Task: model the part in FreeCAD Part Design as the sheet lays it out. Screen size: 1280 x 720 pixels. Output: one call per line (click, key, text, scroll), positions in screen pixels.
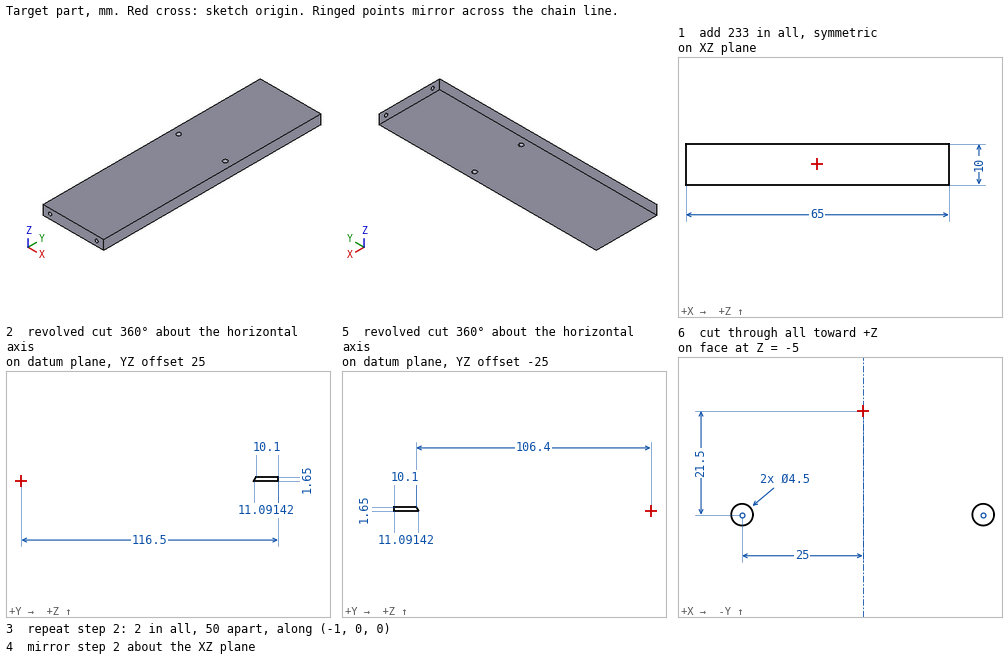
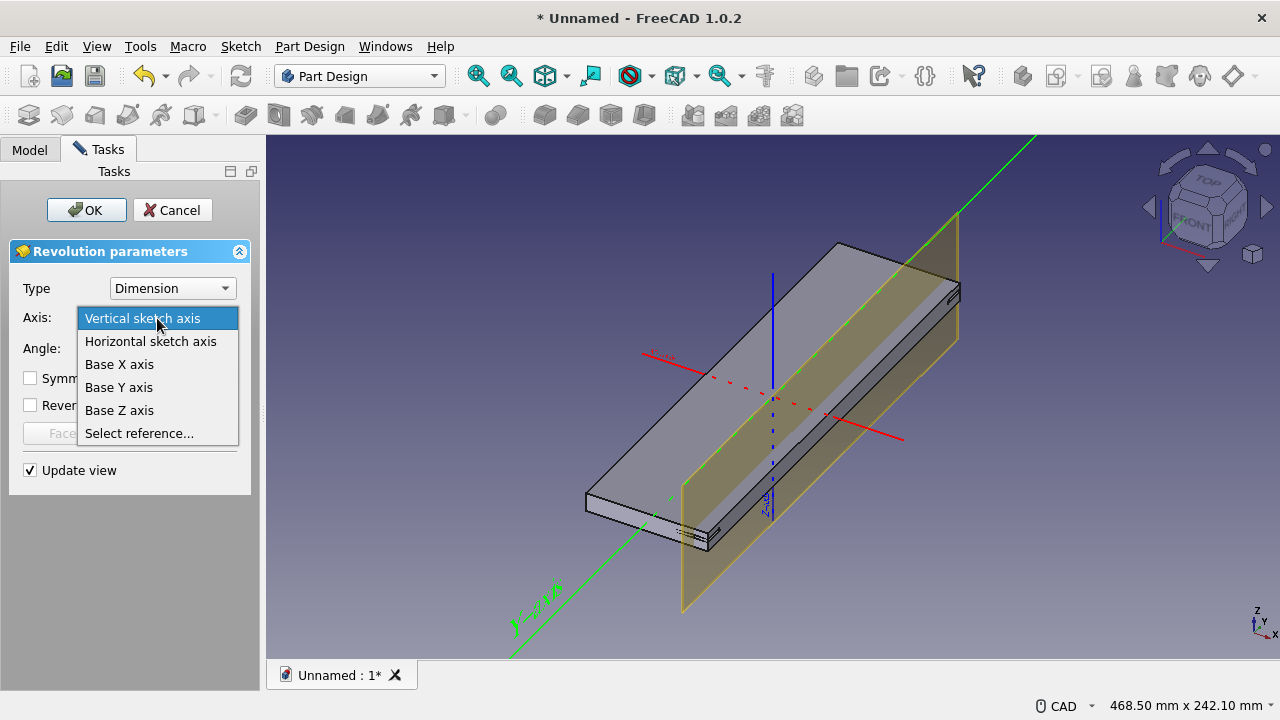
click(156, 342)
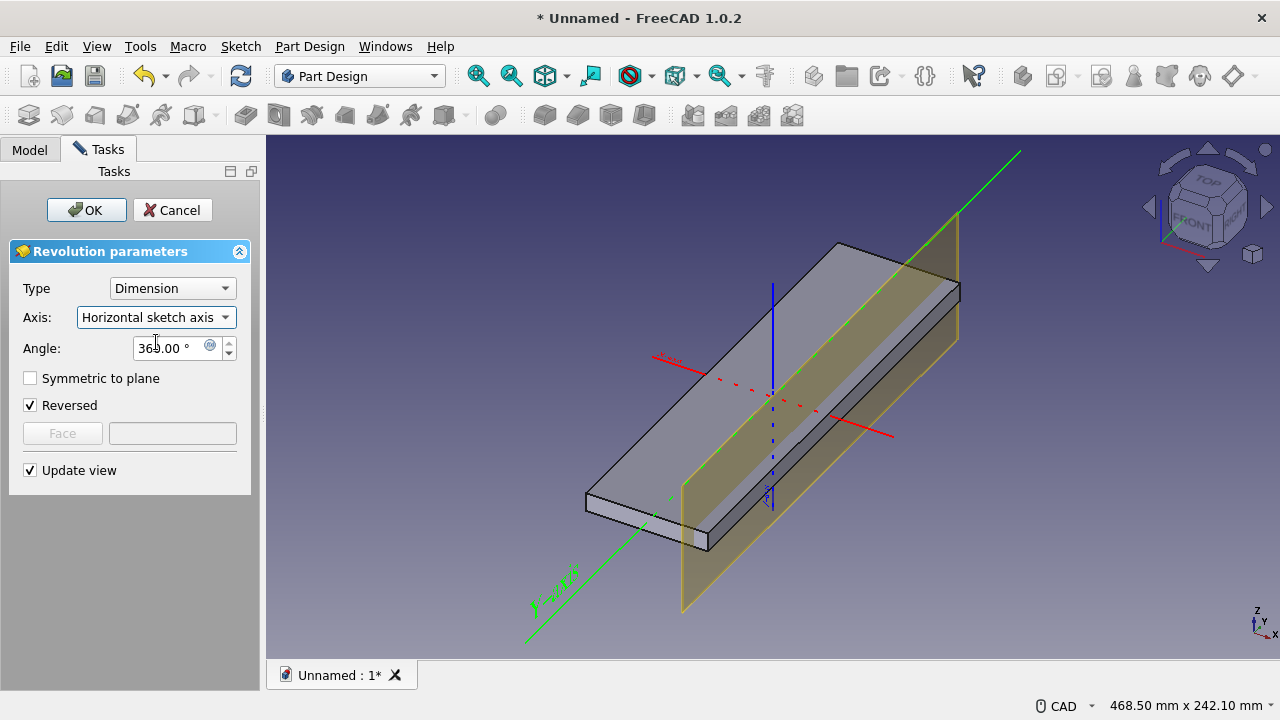
click(87, 210)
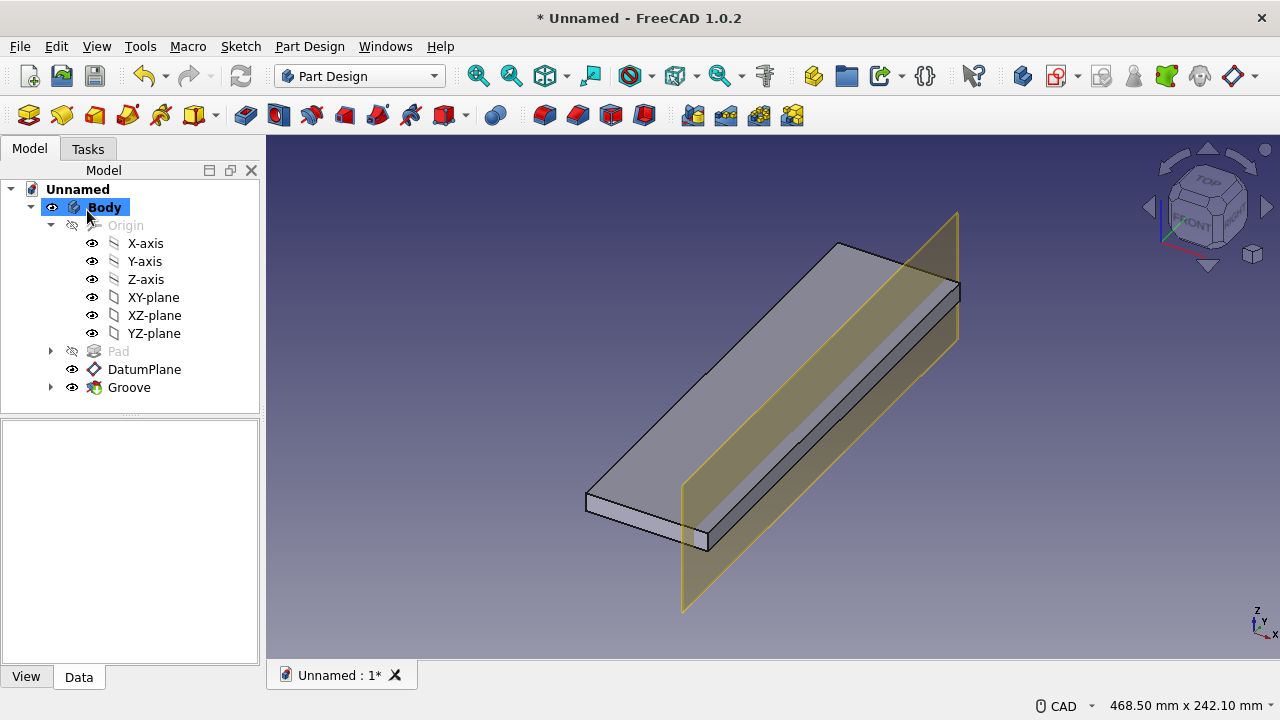
click(117, 369)
key(space)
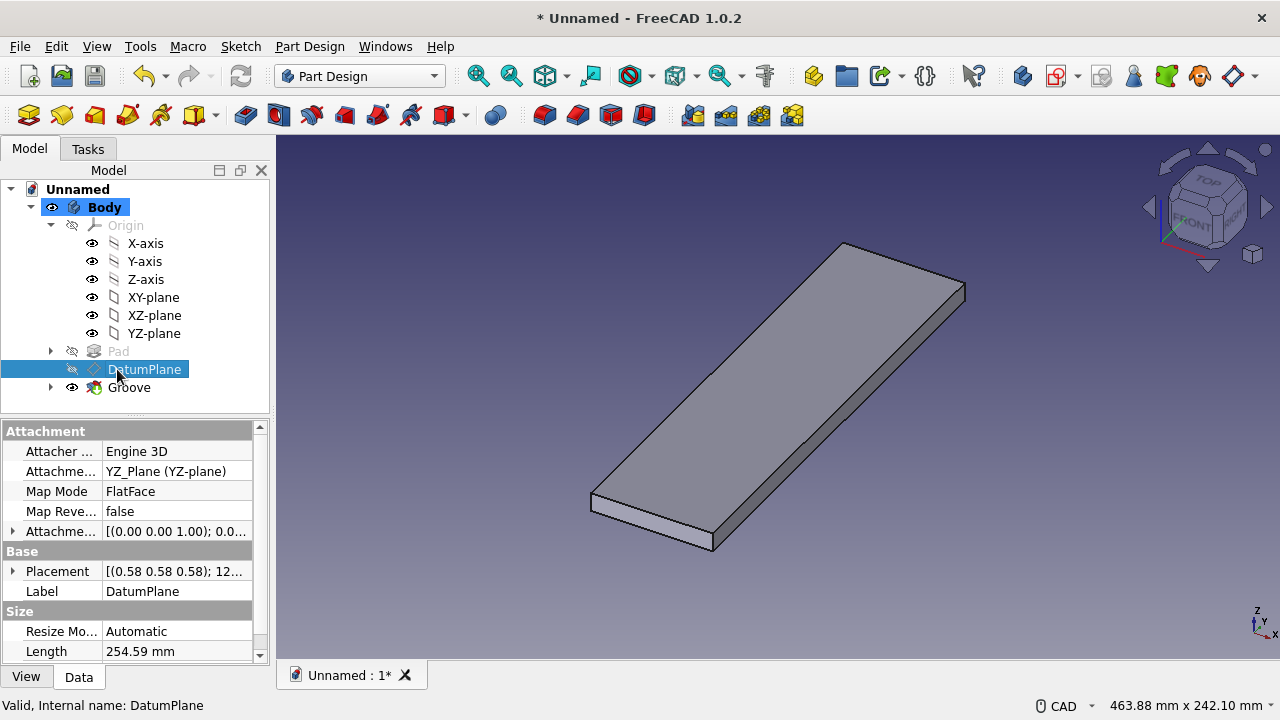
click(117, 387)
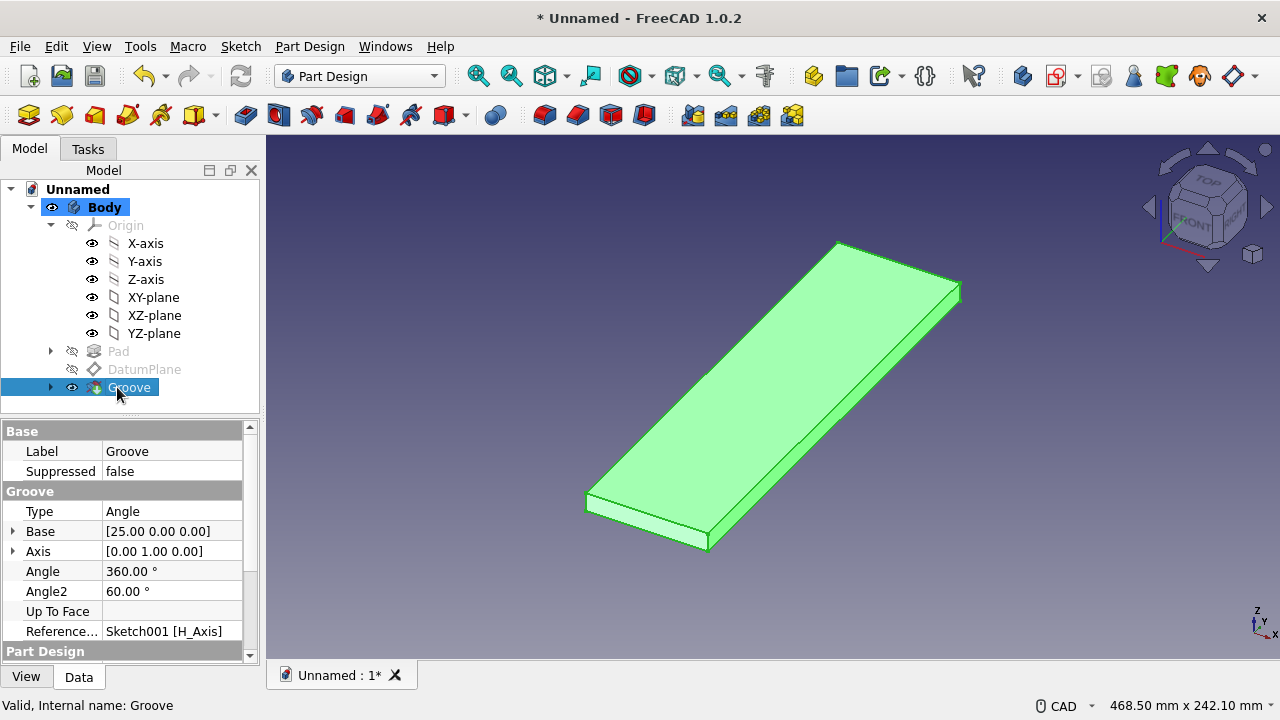
click(726, 116)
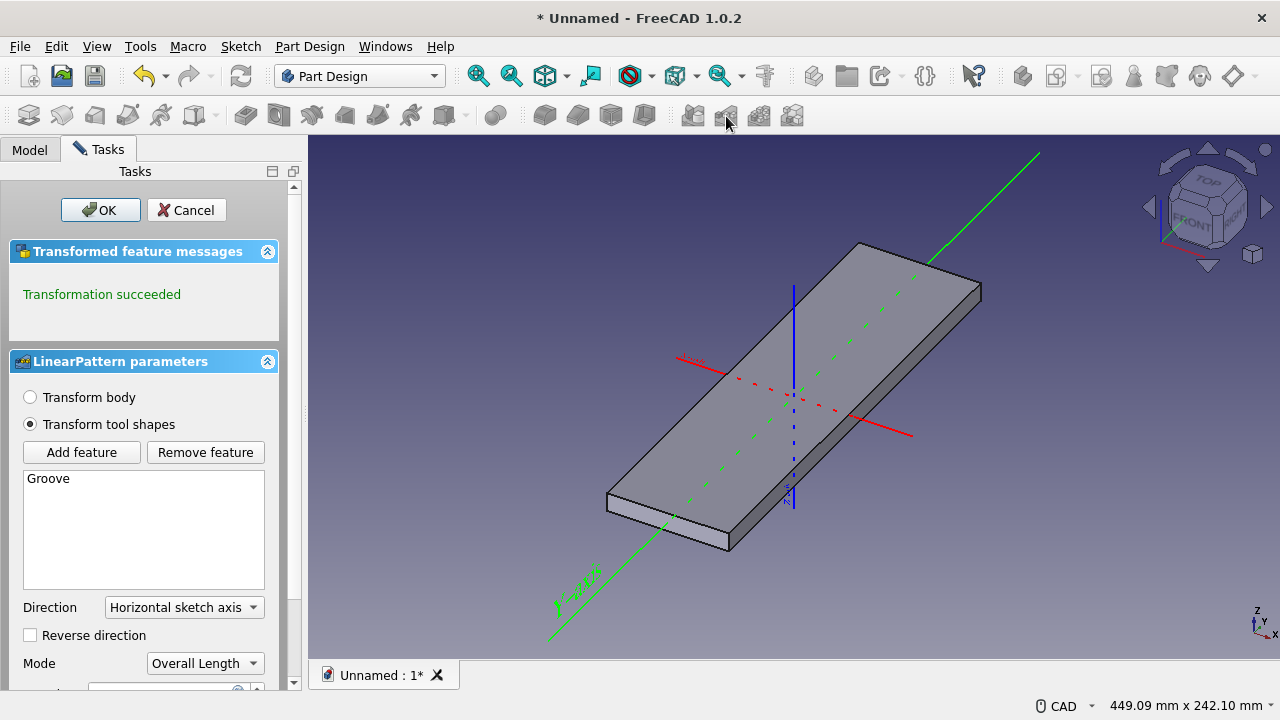
click(185, 608)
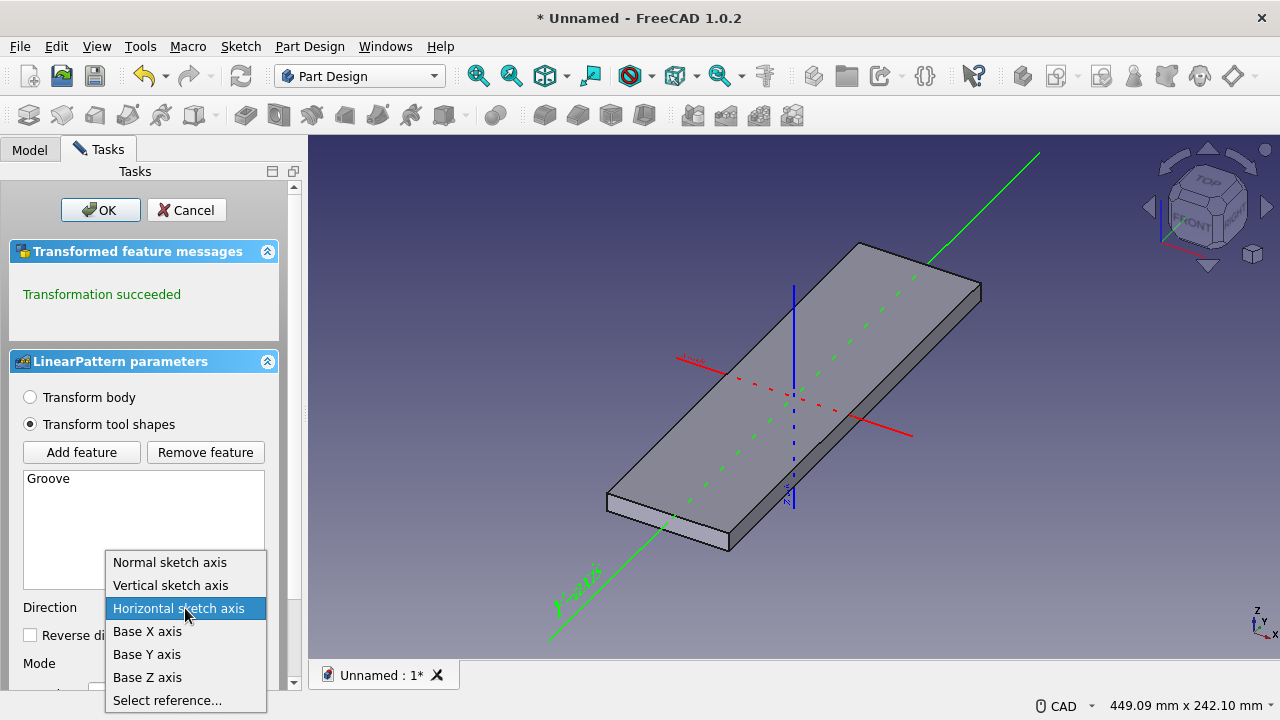
click(184, 632)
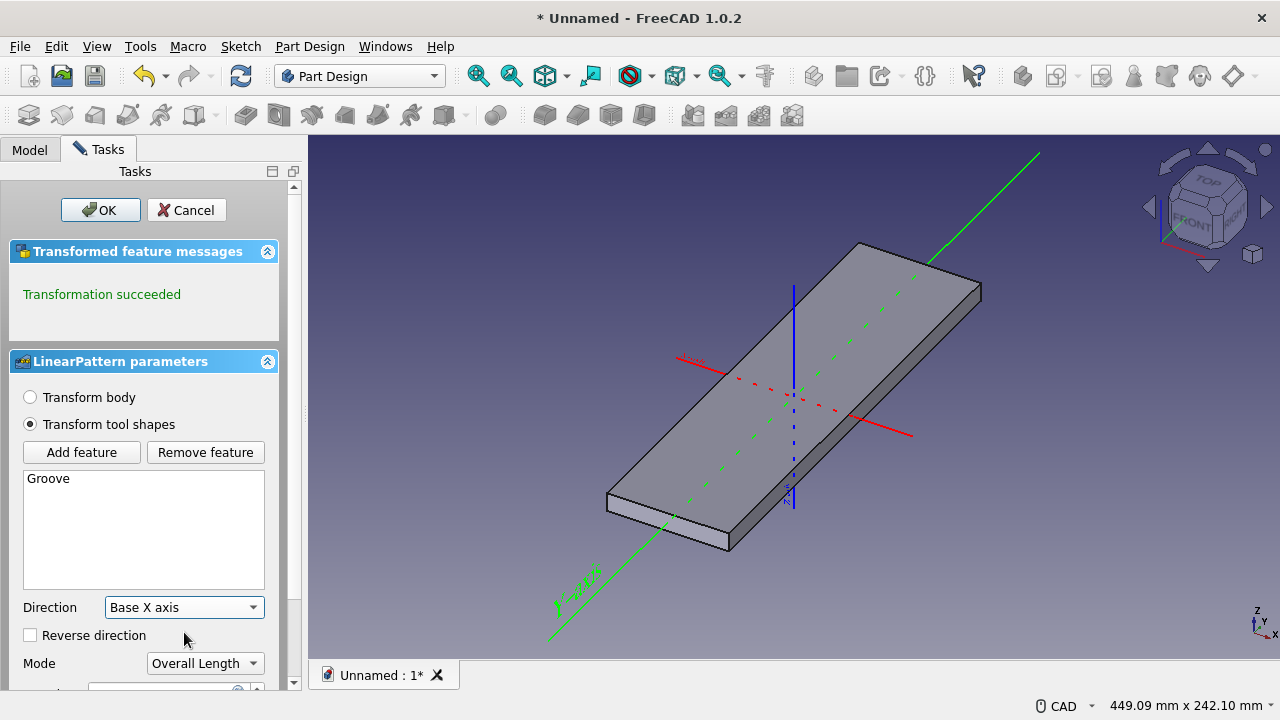
click(206, 664)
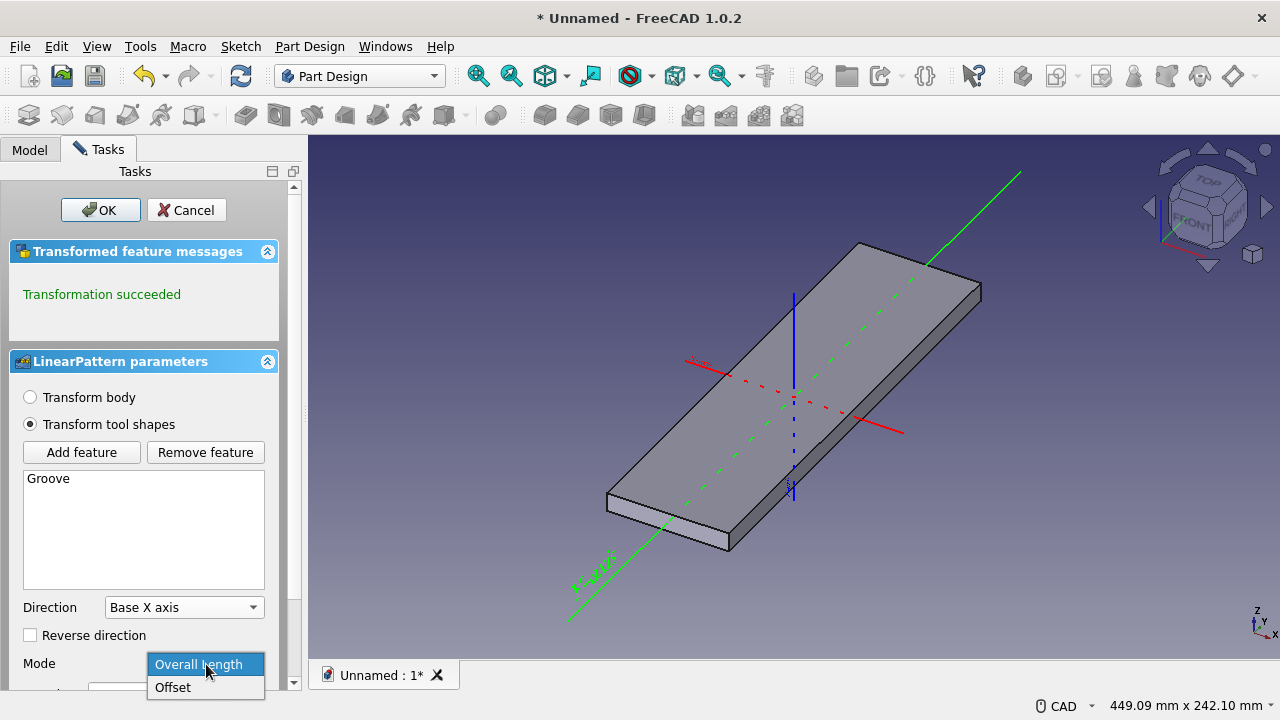
click(204, 688)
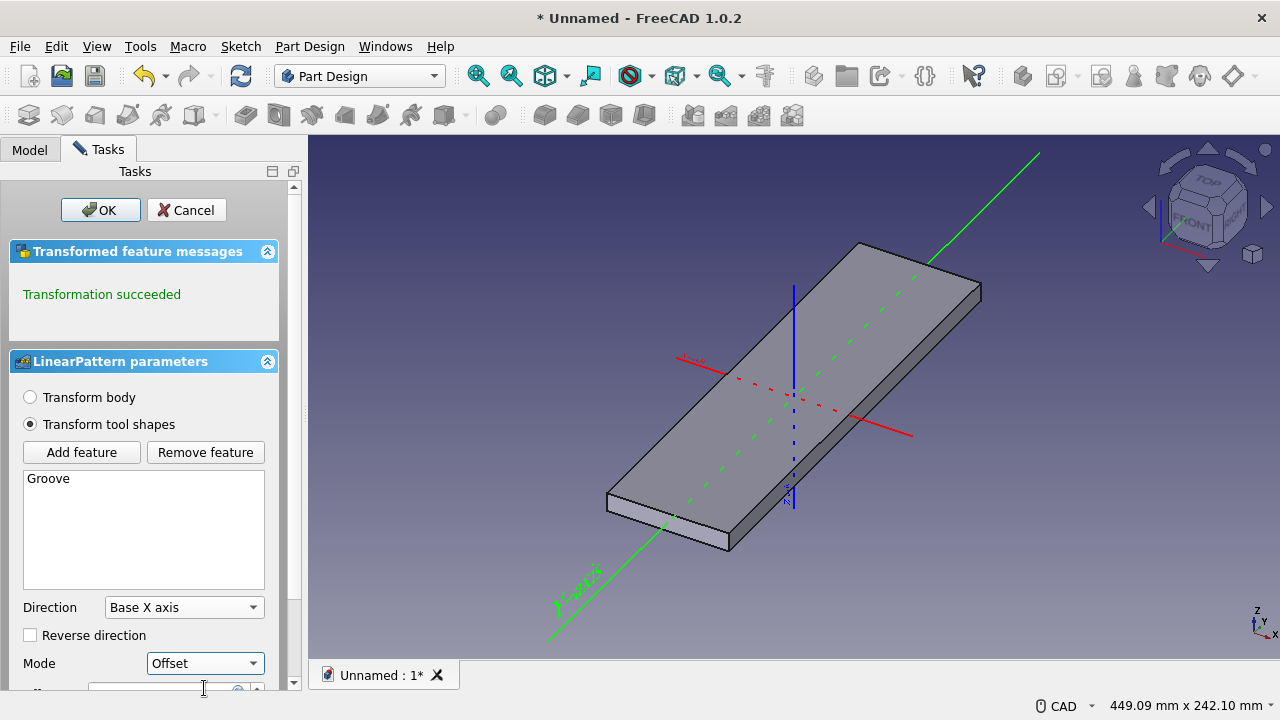
scroll(294, 436, down, 2)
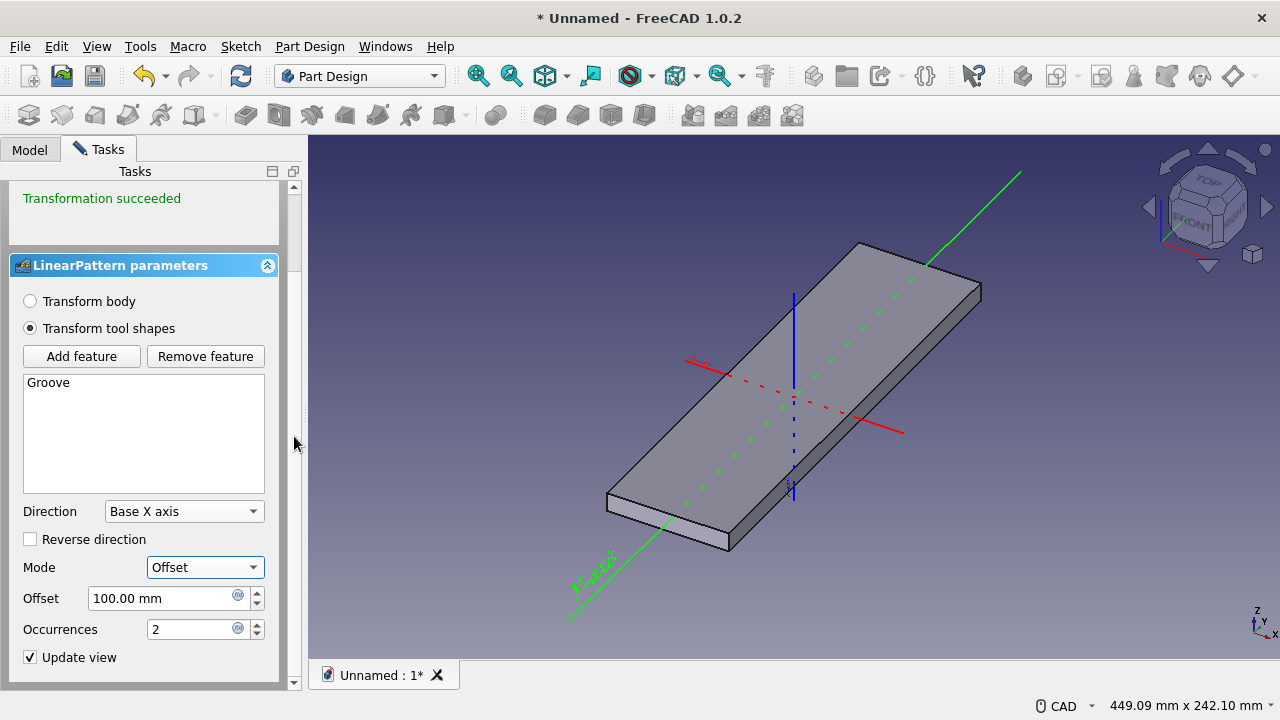
triple_click(170, 598)